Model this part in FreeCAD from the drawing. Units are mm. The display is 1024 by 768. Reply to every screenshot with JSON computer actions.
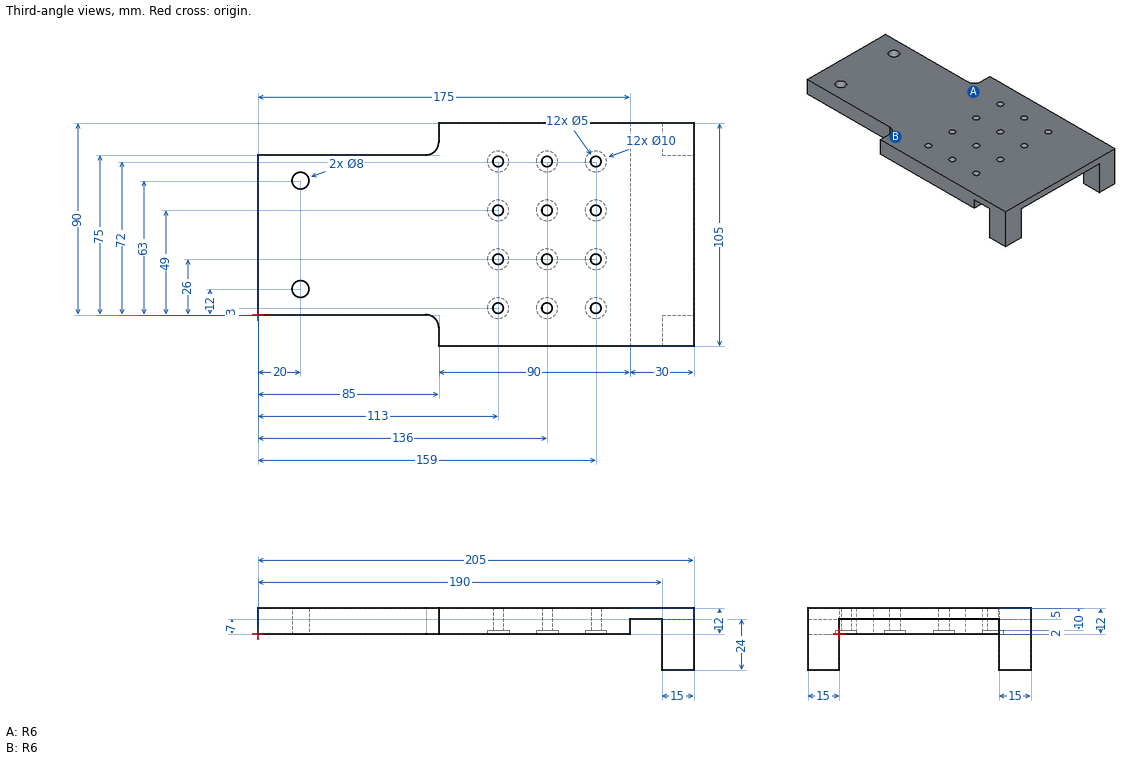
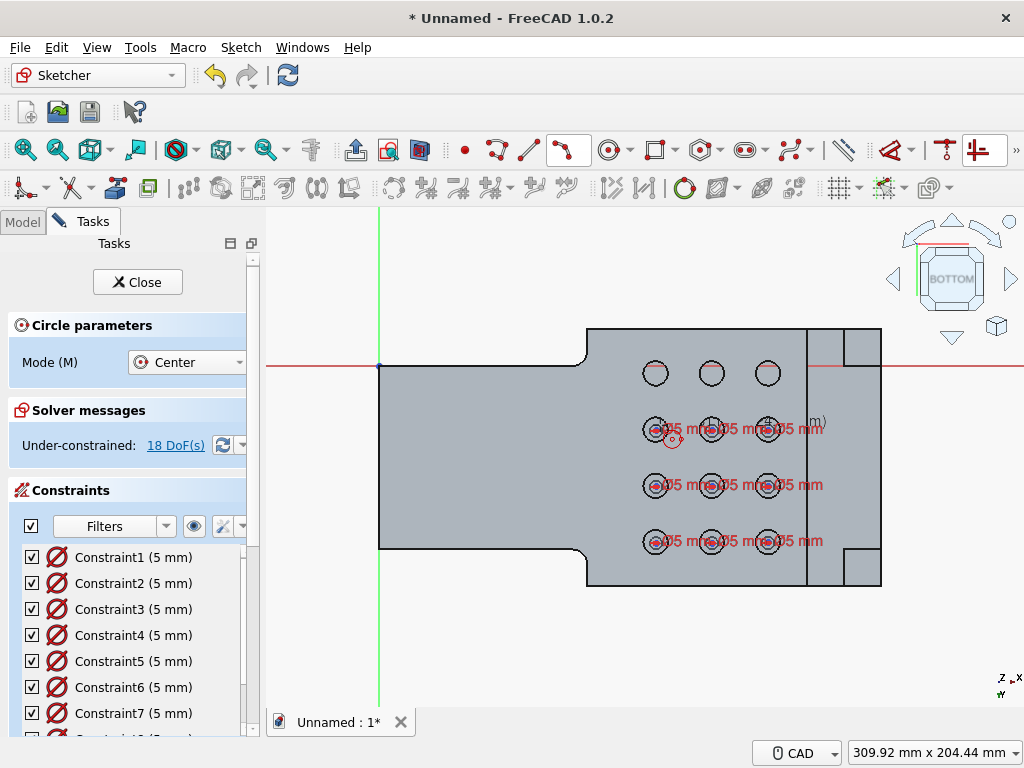
{"action": "scroll", "coordinate": [768, 373], "scroll_direction": "up", "scroll_amount": 7}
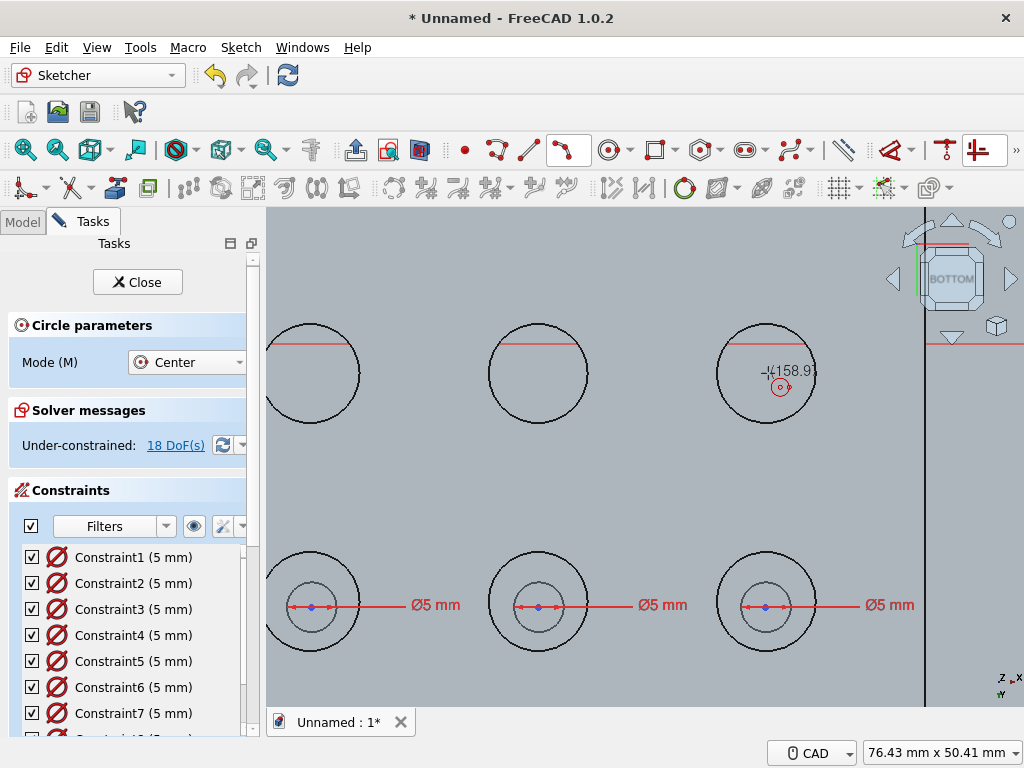
{"action": "left_click", "coordinate": [766, 373]}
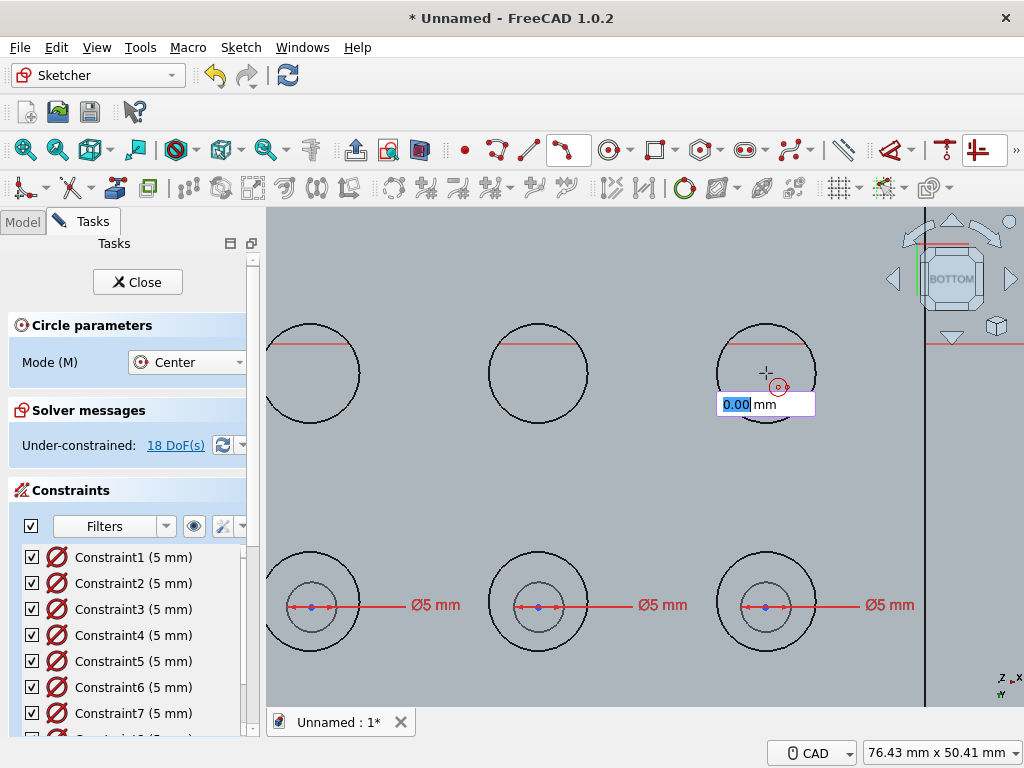
{"action": "scroll", "coordinate": [768, 373], "scroll_direction": "down", "scroll_amount": 7}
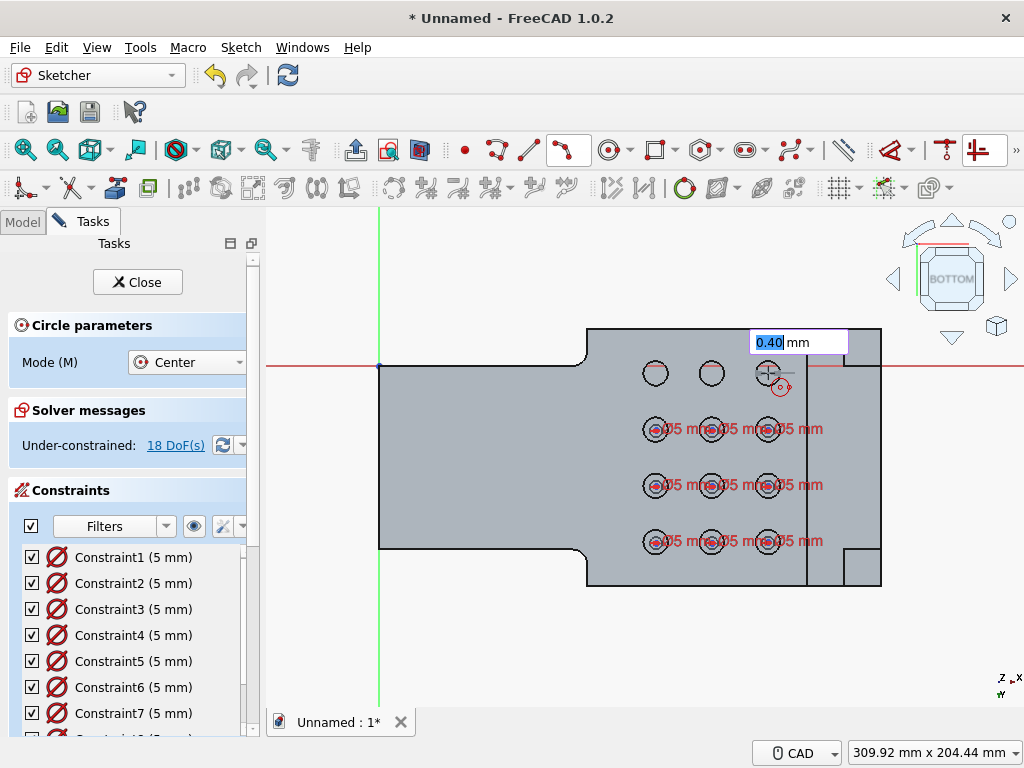
{"action": "scroll", "coordinate": [772, 378], "scroll_direction": "up", "scroll_amount": 2}
{"action": "mouse_move", "coordinate": [772, 377]}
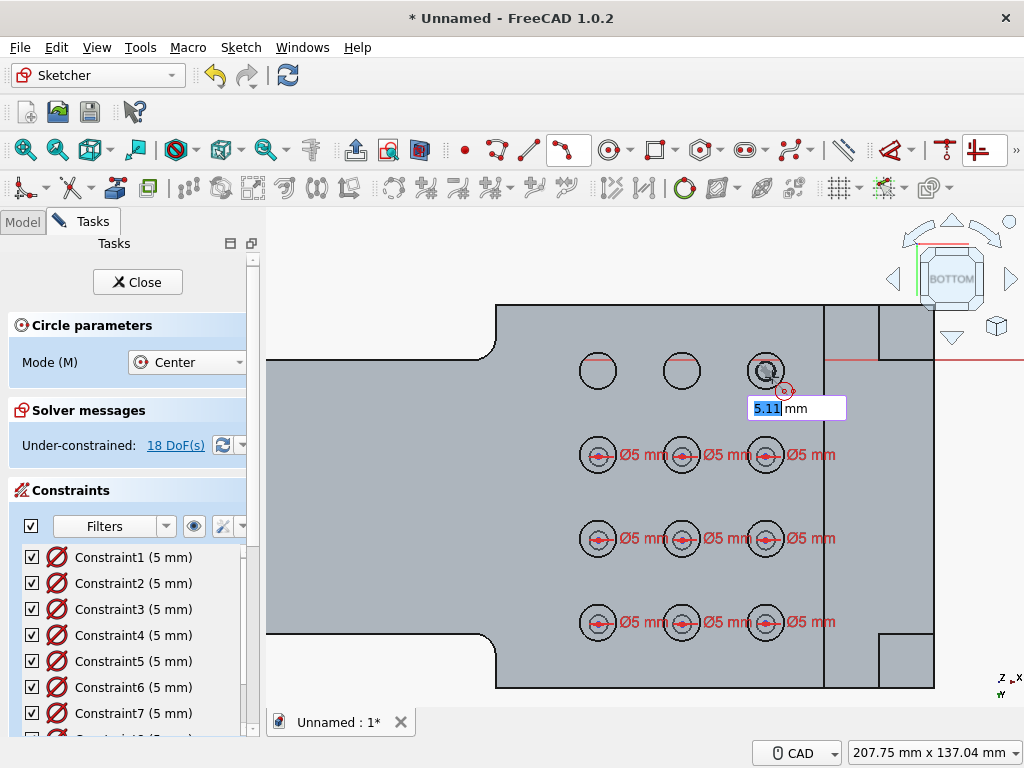
{"action": "type", "text": "5"}
{"action": "key", "text": "Return"}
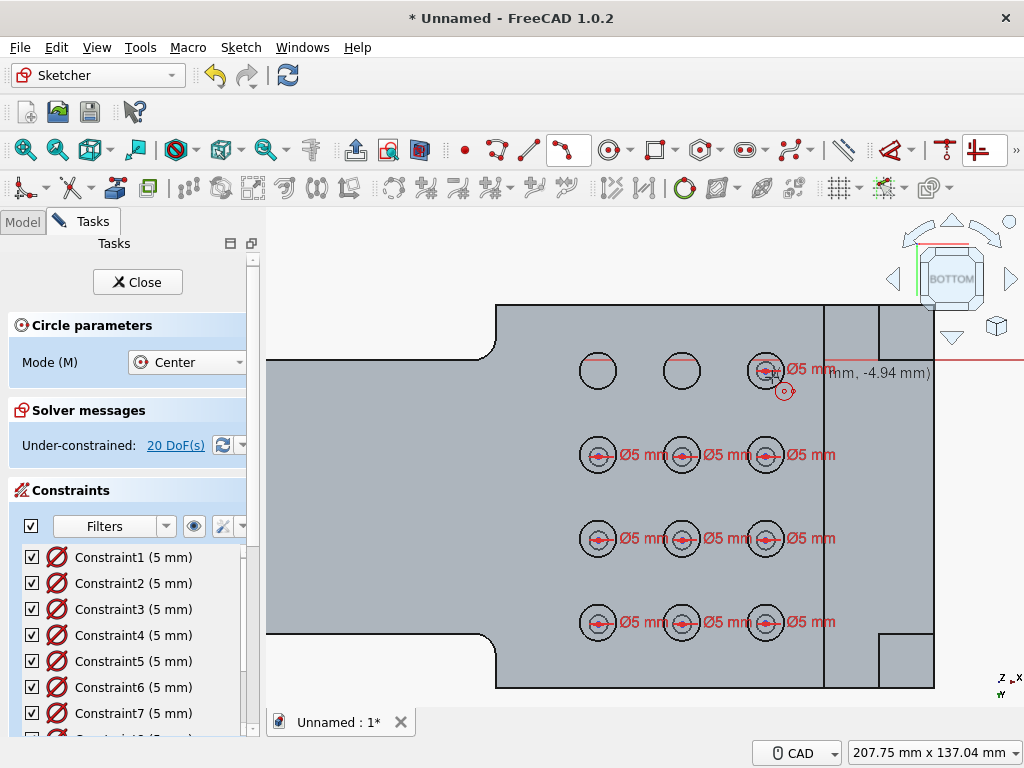
{"action": "scroll", "coordinate": [682, 371], "scroll_direction": "up", "scroll_amount": 5}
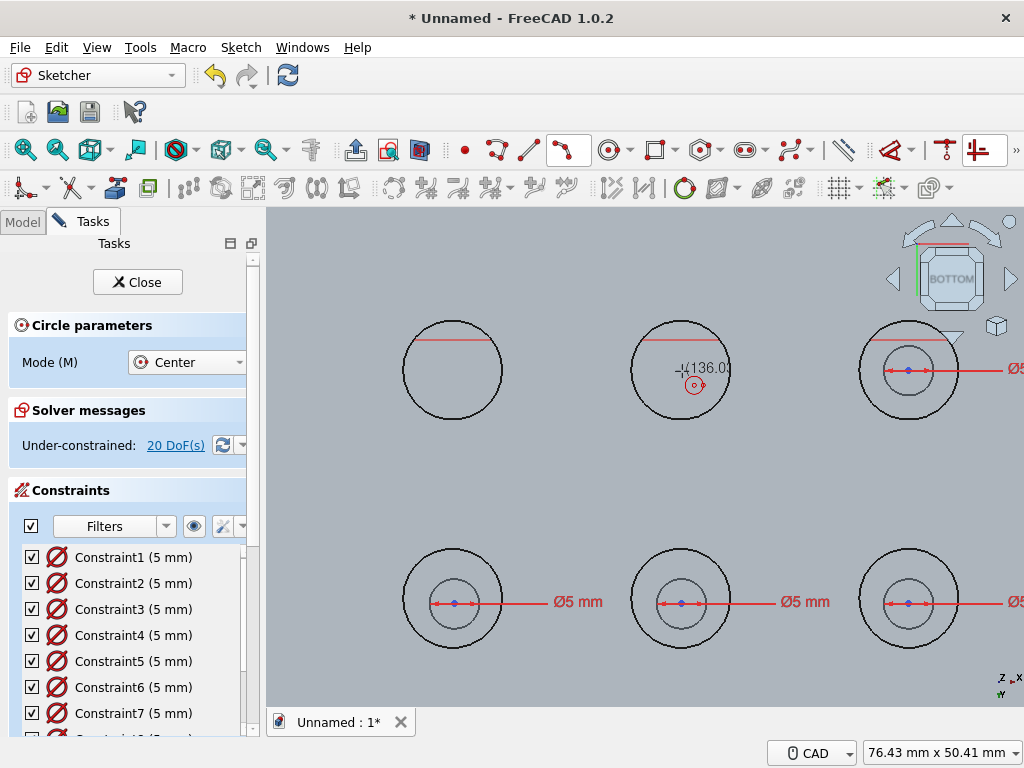
{"action": "left_click", "coordinate": [681, 370]}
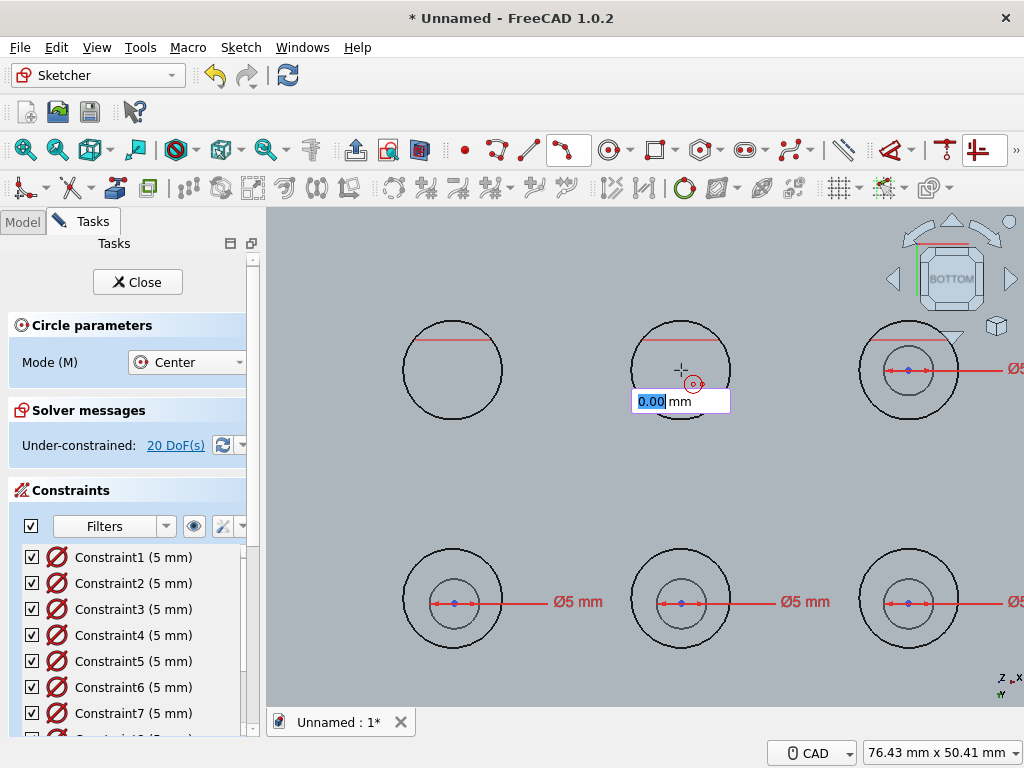
{"action": "scroll", "coordinate": [722, 374], "scroll_direction": "down", "scroll_amount": 7}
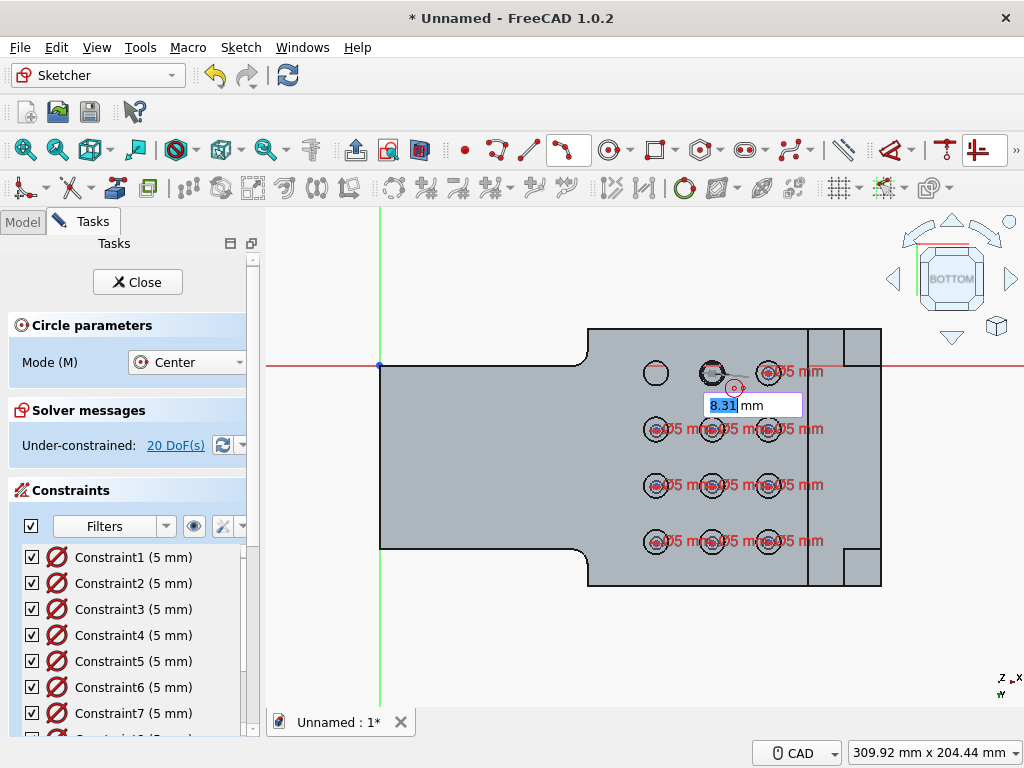
{"action": "scroll", "coordinate": [717, 378], "scroll_direction": "up", "scroll_amount": 2}
{"action": "mouse_move", "coordinate": [716, 377]}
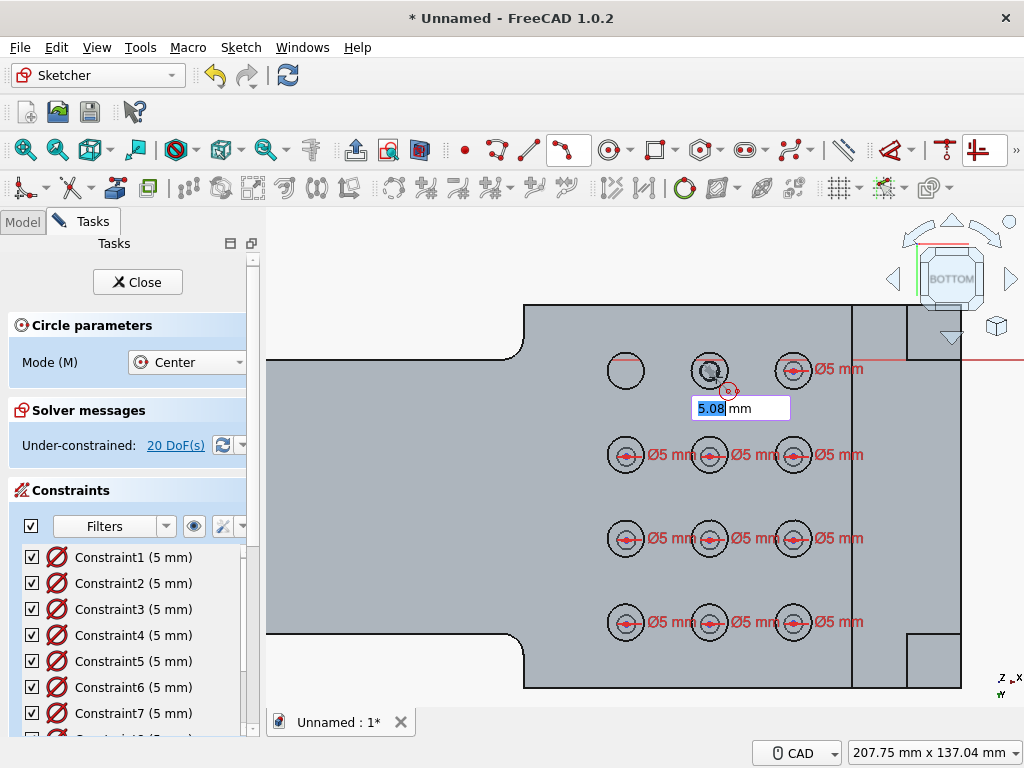
{"action": "type", "text": "5"}
{"action": "key", "text": "Return"}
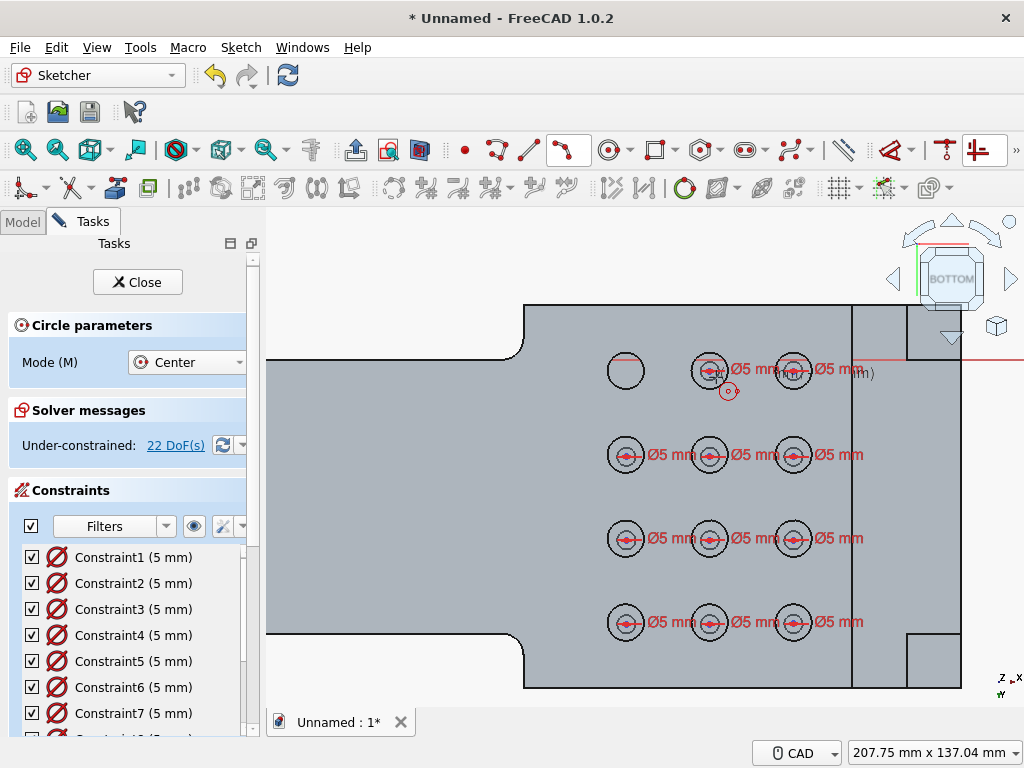
{"action": "scroll", "coordinate": [626, 371], "scroll_direction": "up", "scroll_amount": 5}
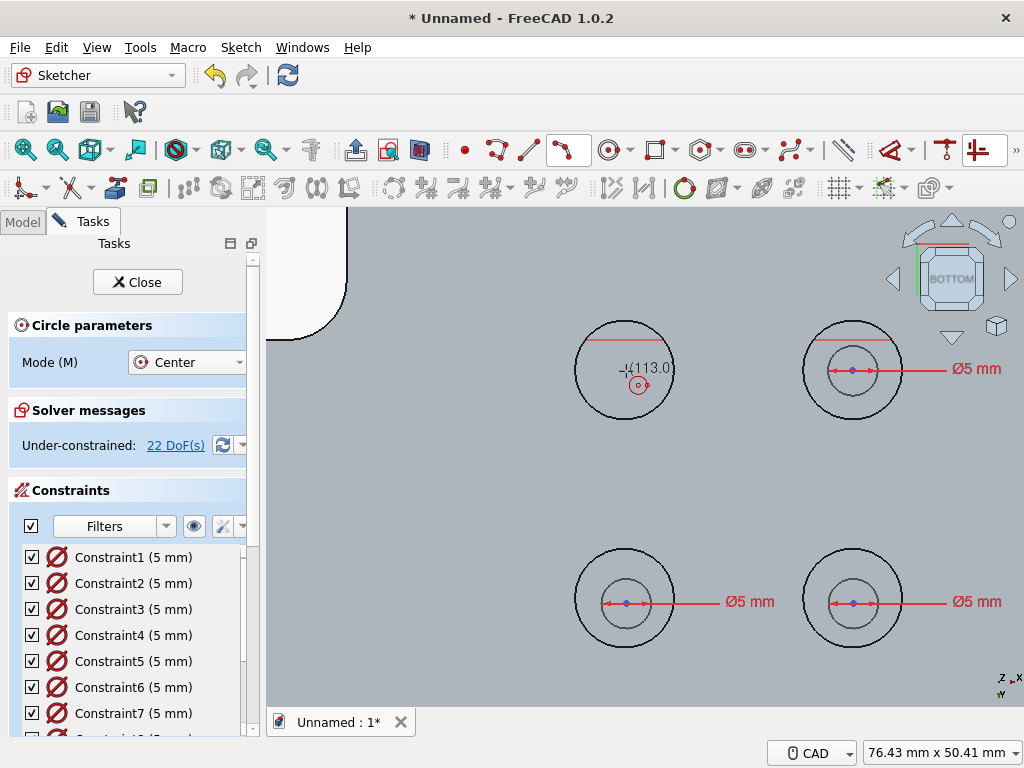
{"action": "left_click", "coordinate": [625, 370]}